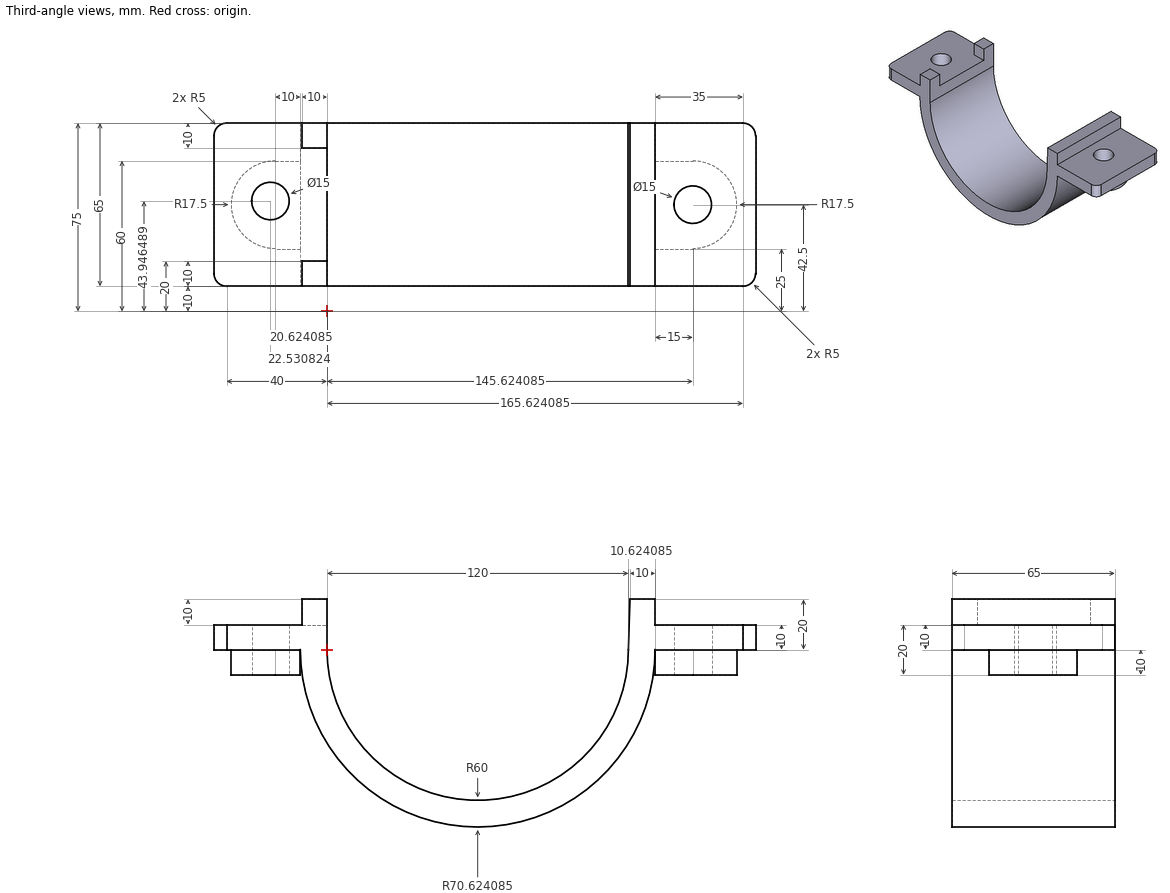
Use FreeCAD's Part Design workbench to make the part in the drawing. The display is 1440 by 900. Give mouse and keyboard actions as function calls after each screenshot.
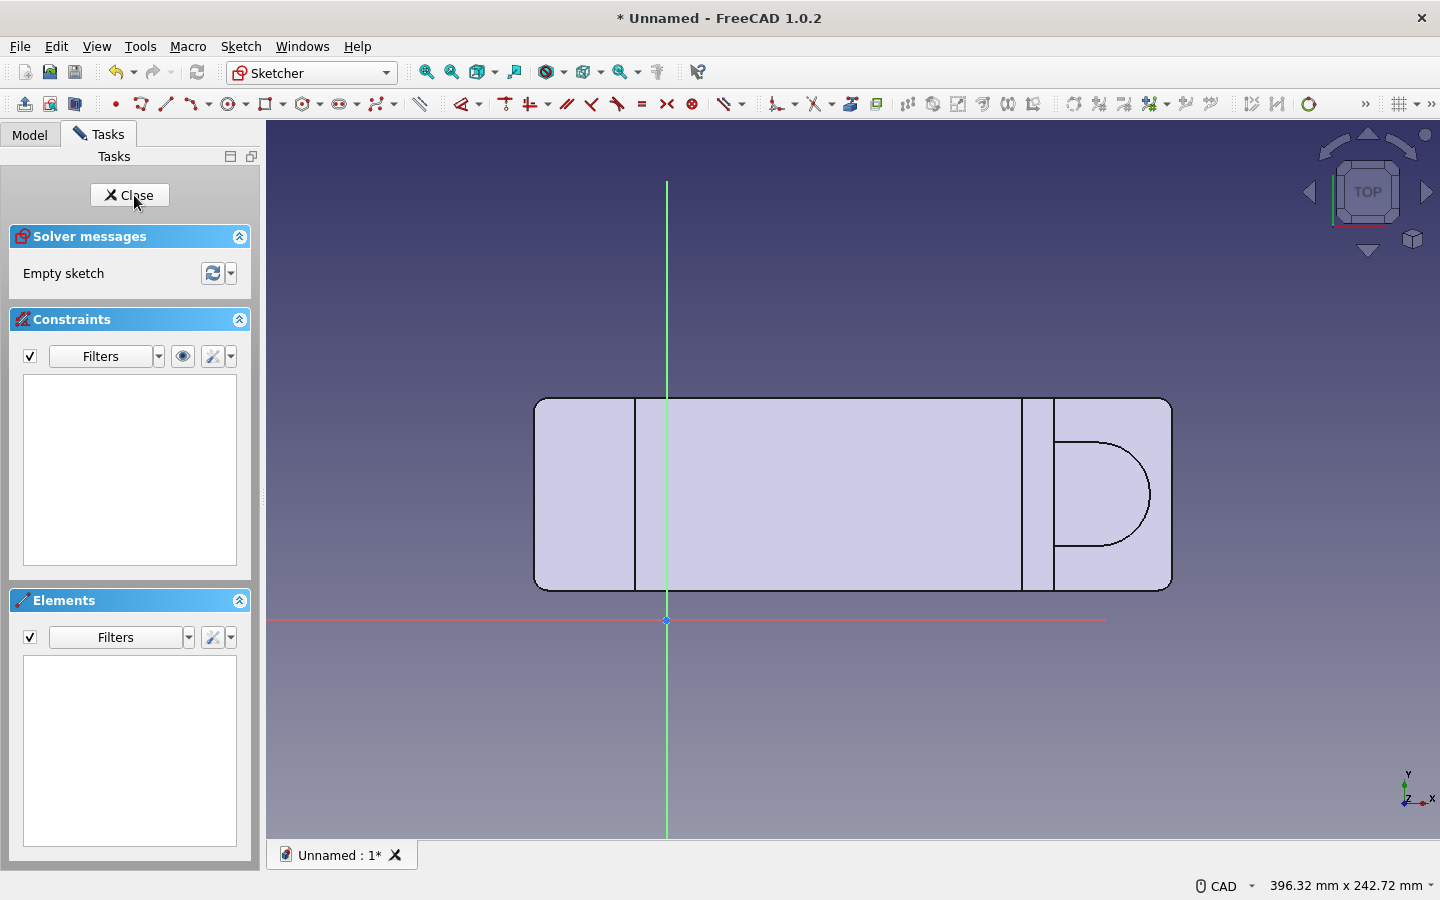
scroll(509, 562, up, 5)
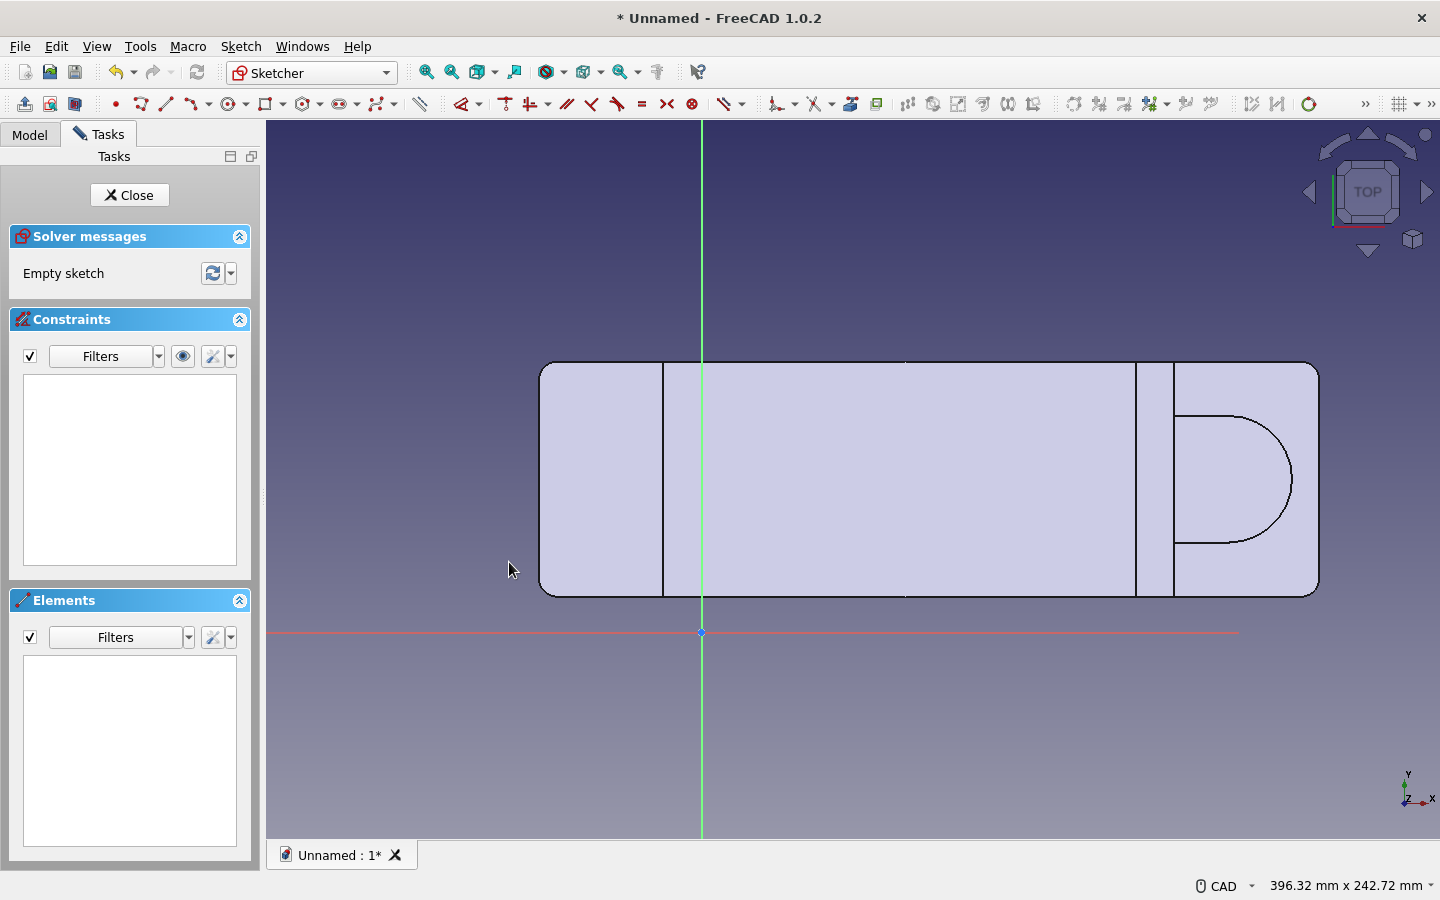
key(g)
key(m)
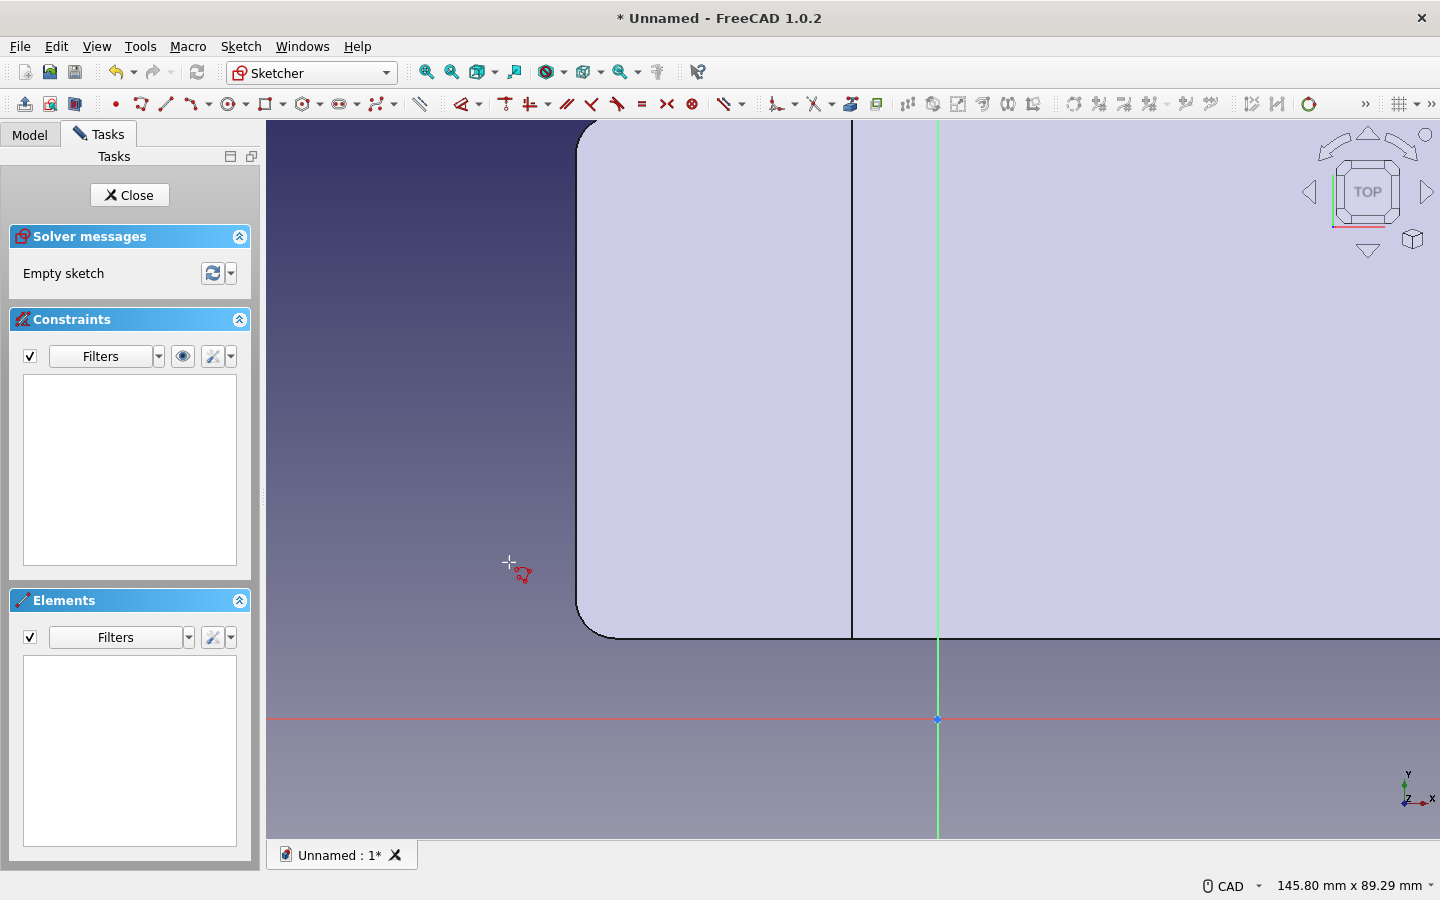
click(772, 236)
click(852, 236)
click(852, 518)
click(772, 518)
right_click(772, 518)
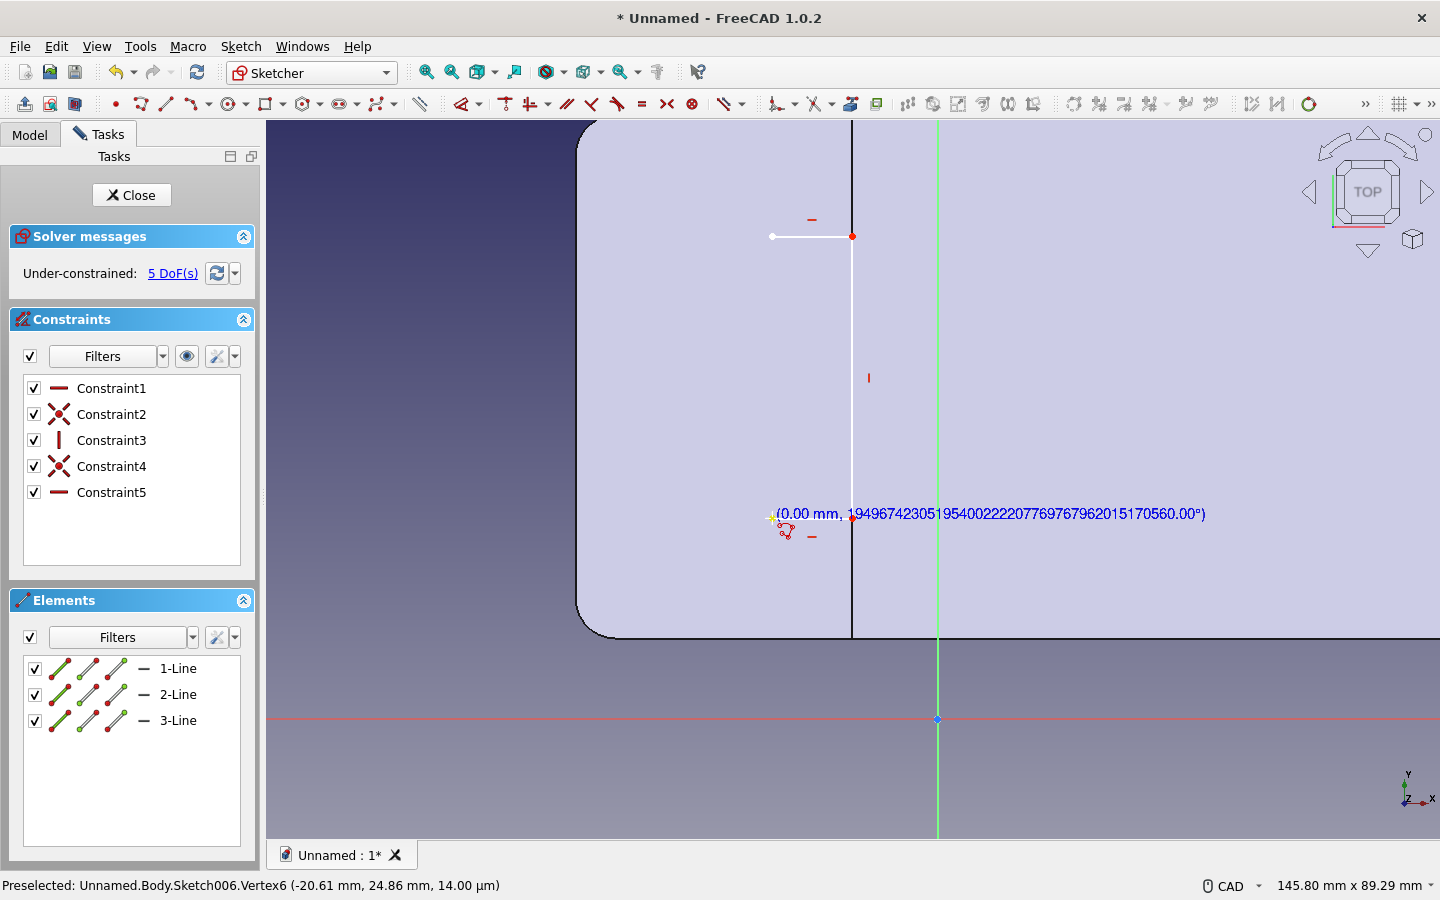
click(190, 104)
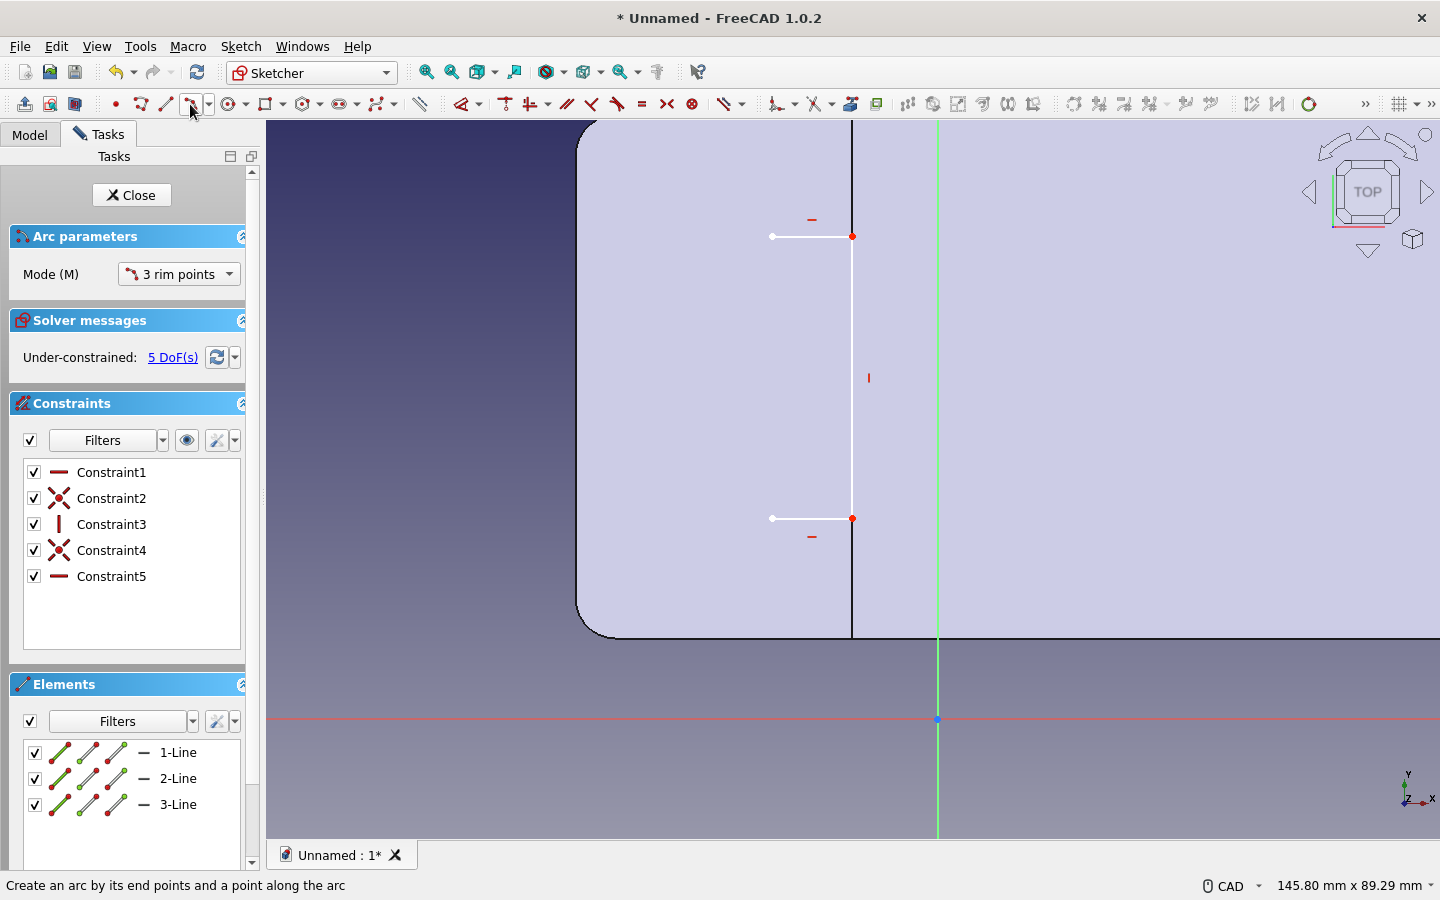
click(772, 519)
click(772, 237)
click(631, 377)
key(Escape)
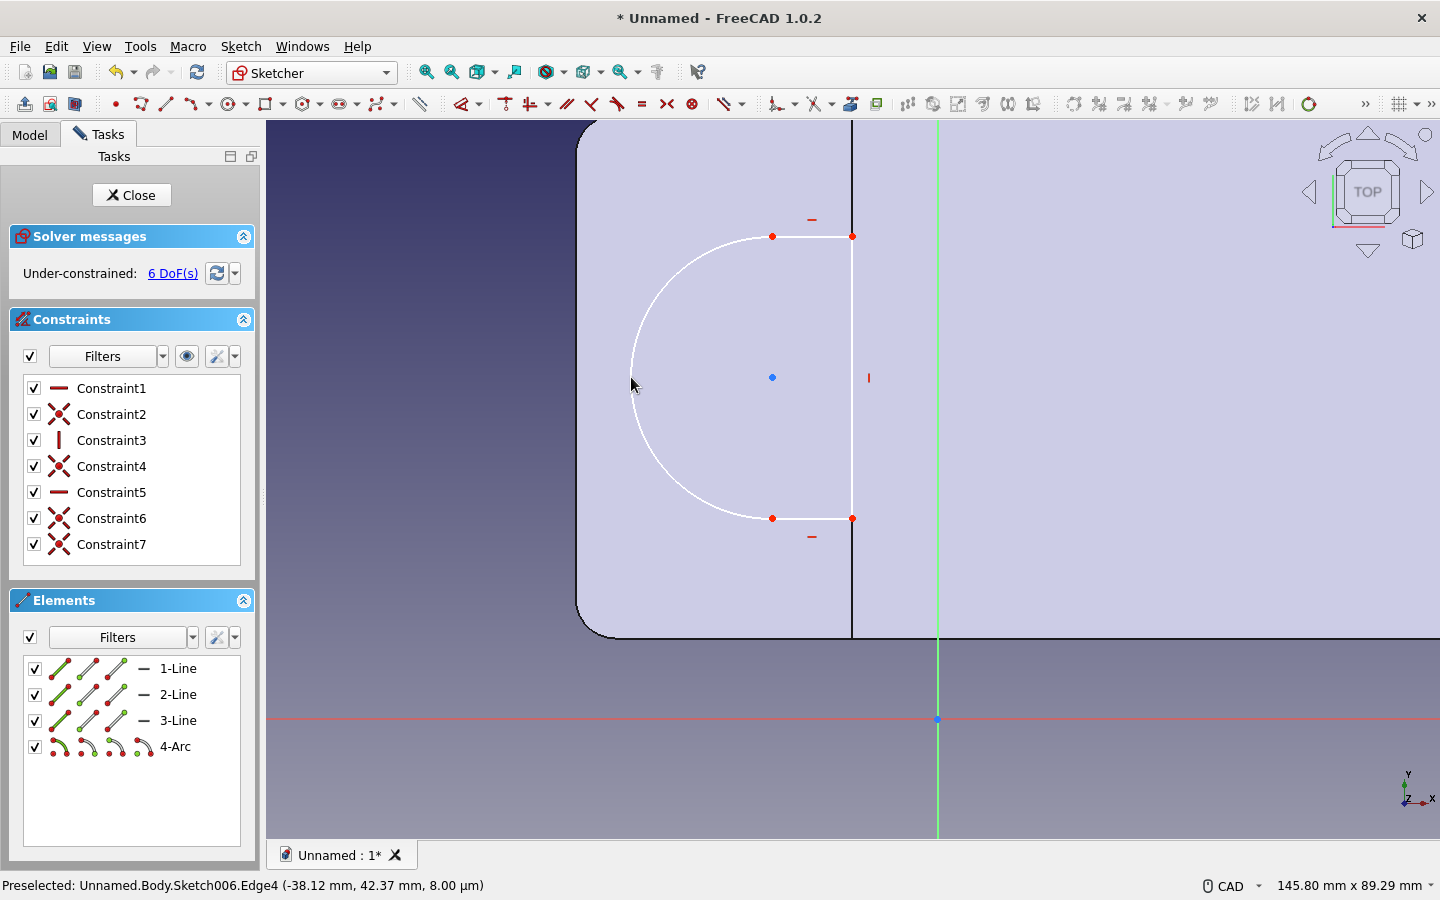
click(796, 237)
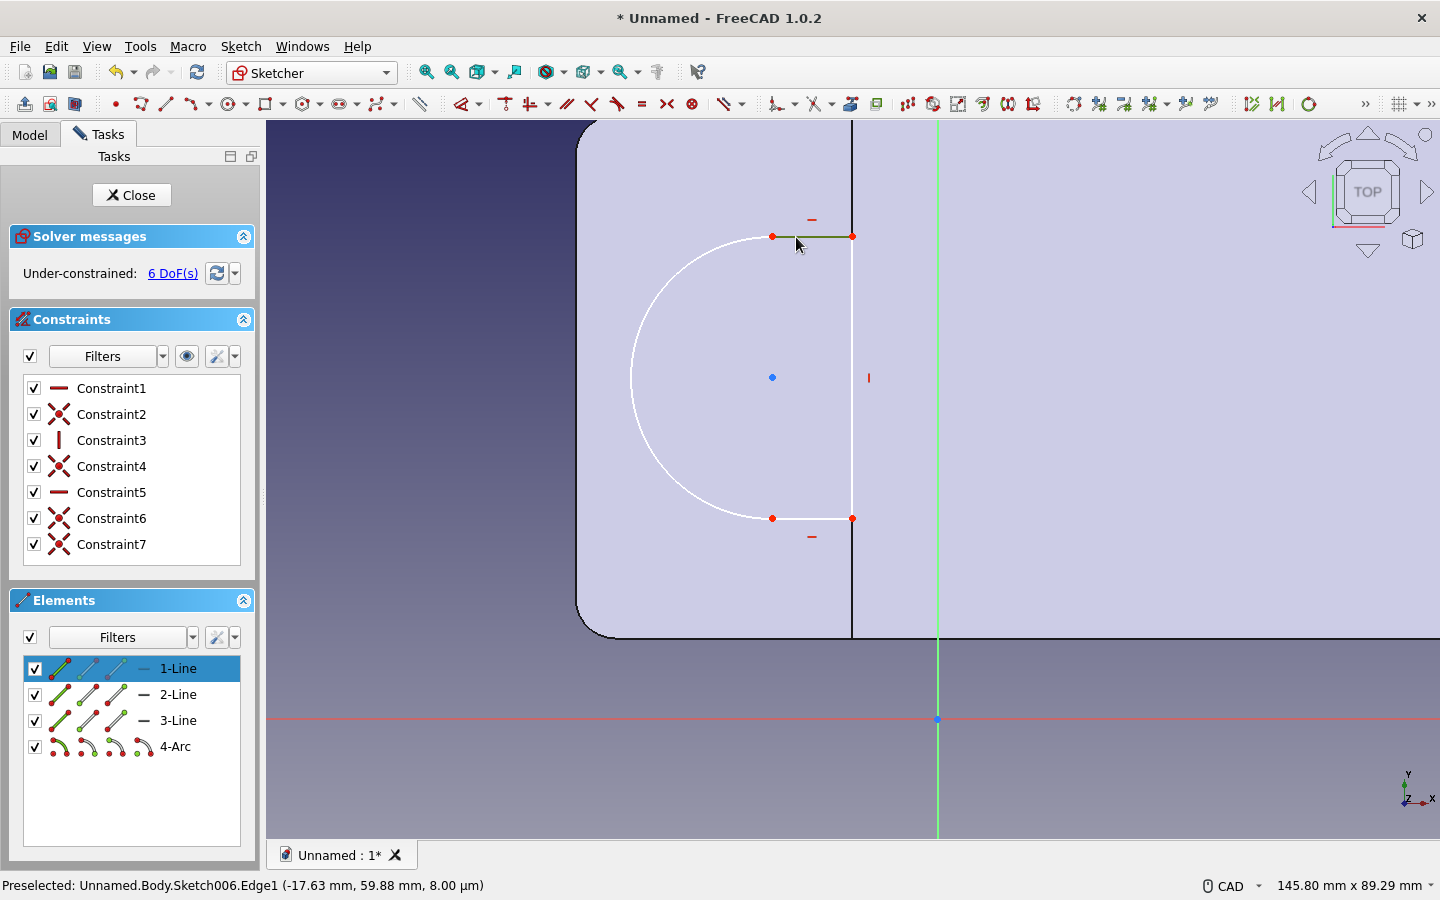
click(658, 295)